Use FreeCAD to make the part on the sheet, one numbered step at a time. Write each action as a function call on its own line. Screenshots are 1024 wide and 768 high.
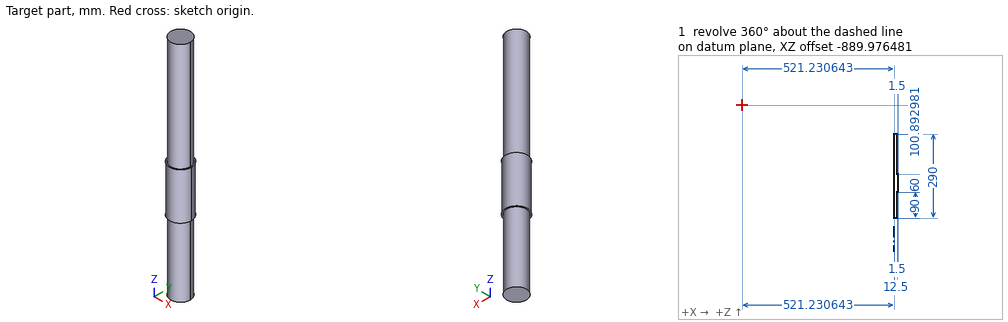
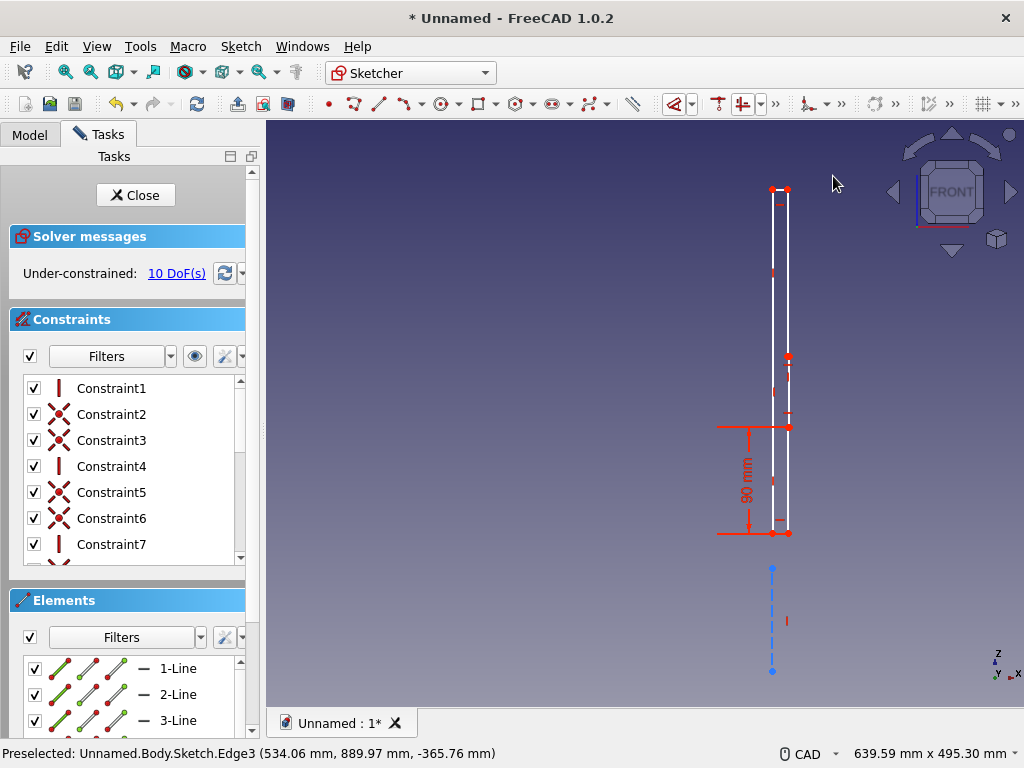
click(789, 399)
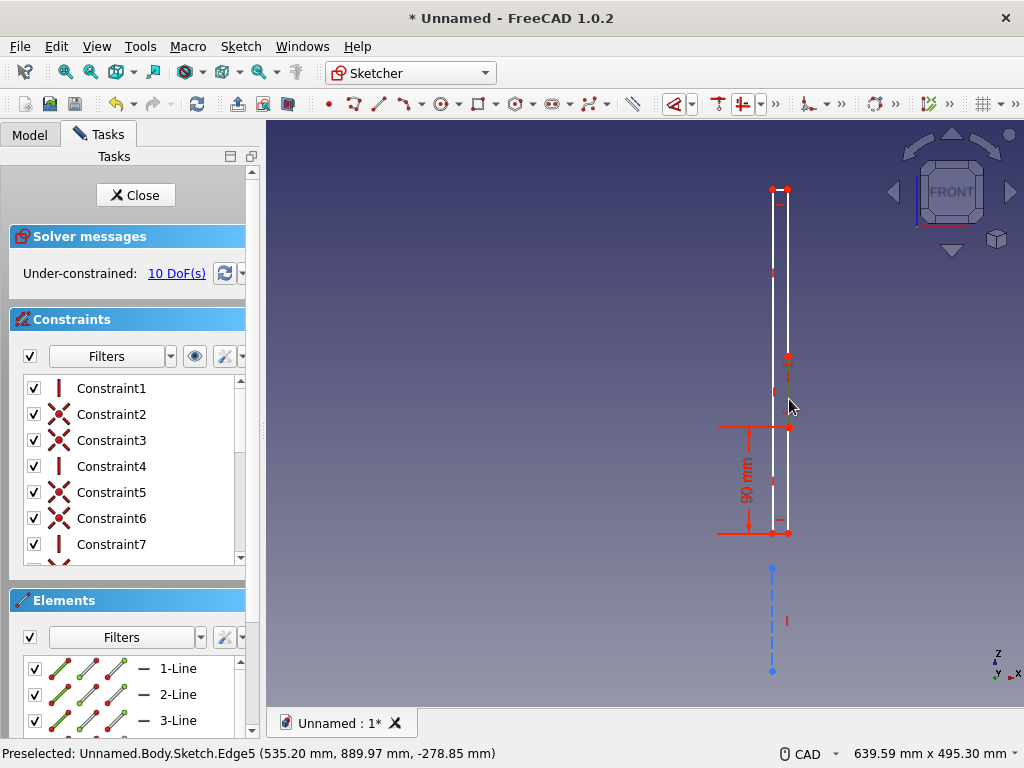
key(i)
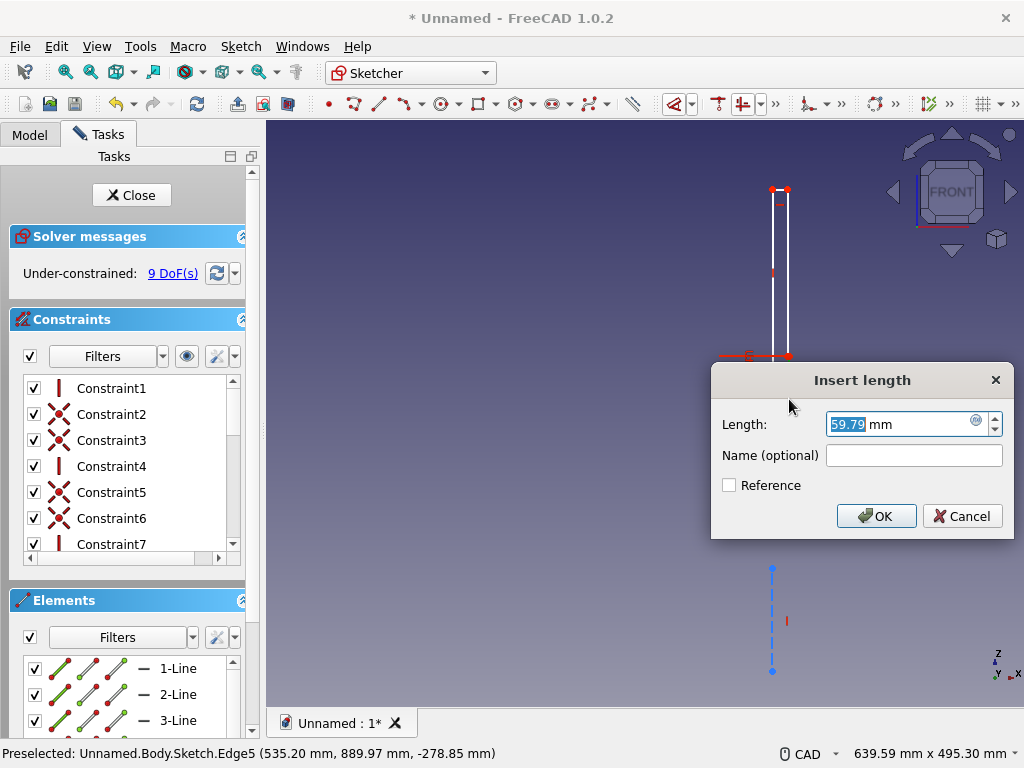
text(60)
key(Return)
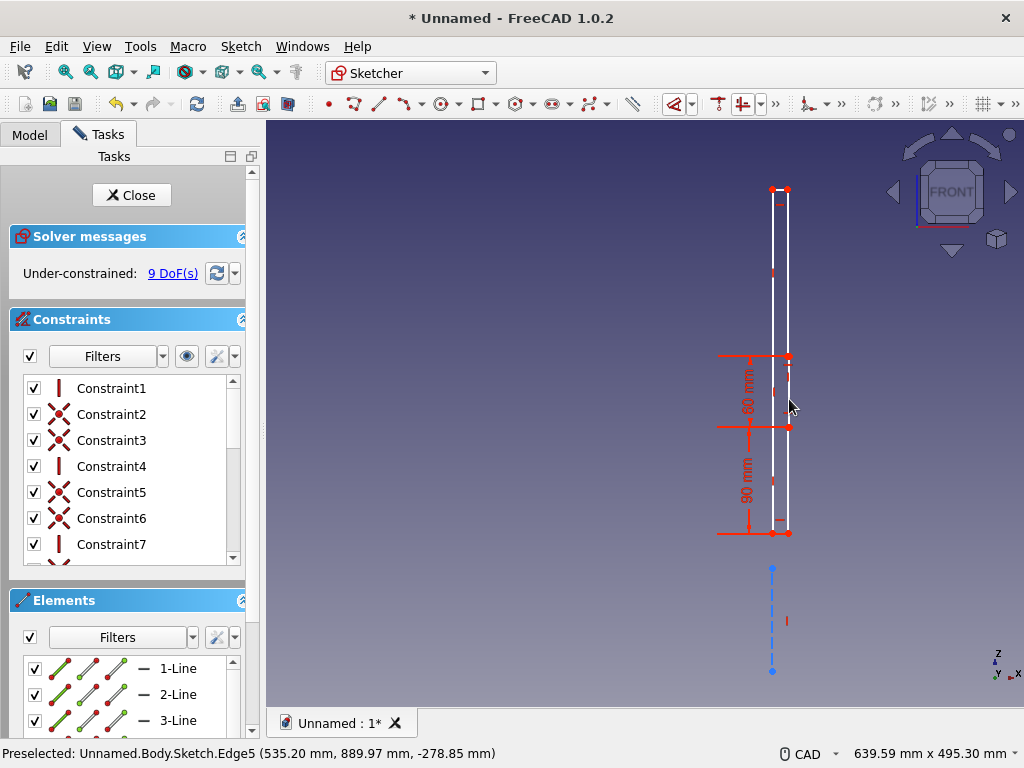
click(773, 293)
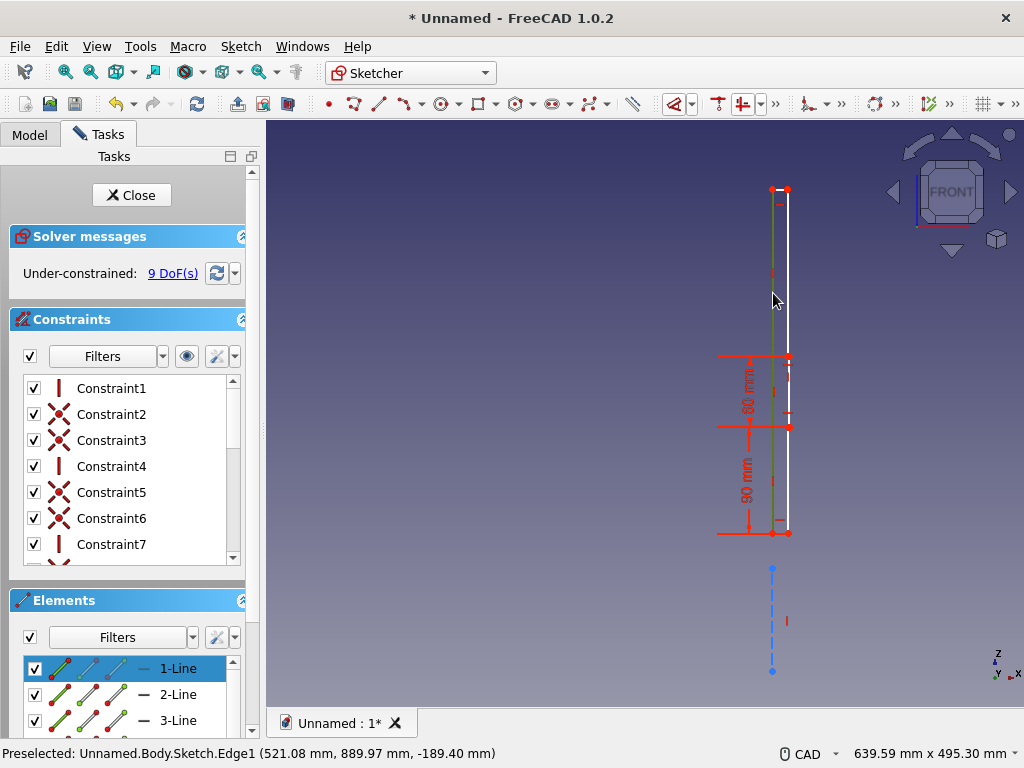
key(i)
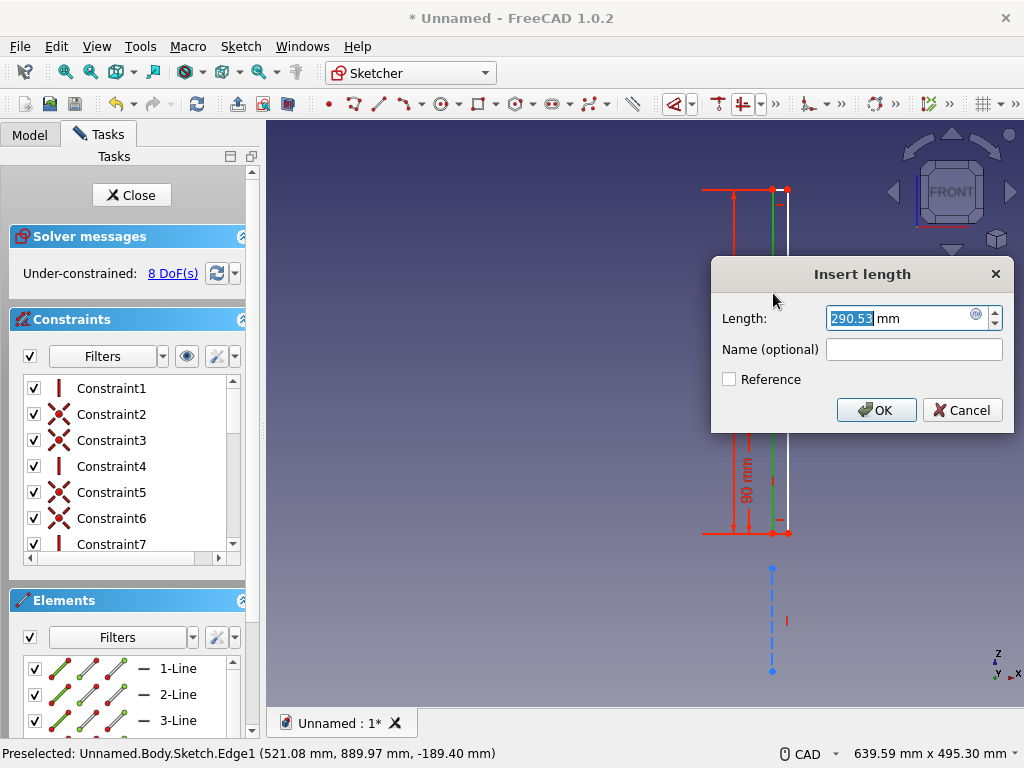
text(290)
key(Return)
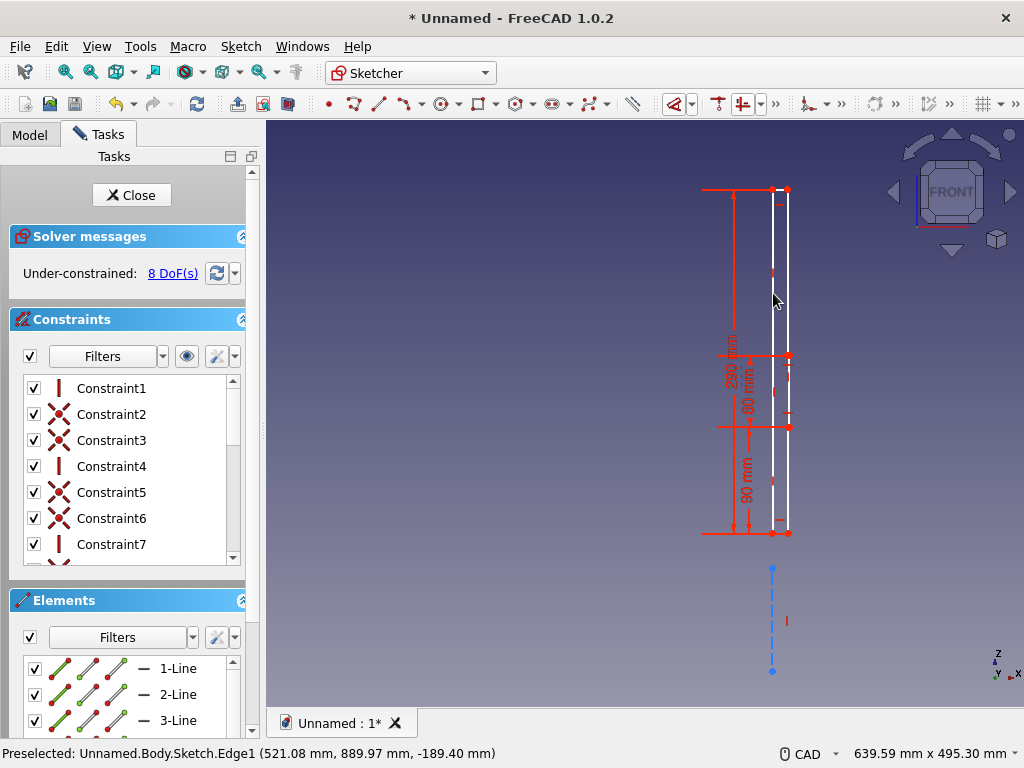
scroll(789, 427, up, 16)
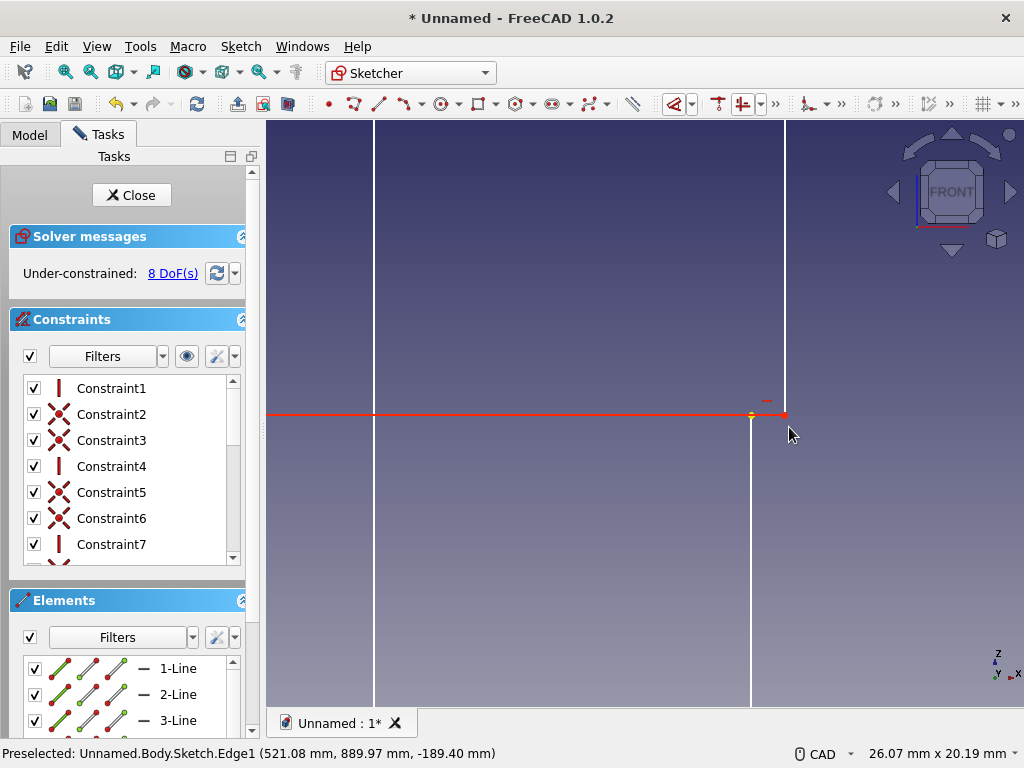
click(768, 415)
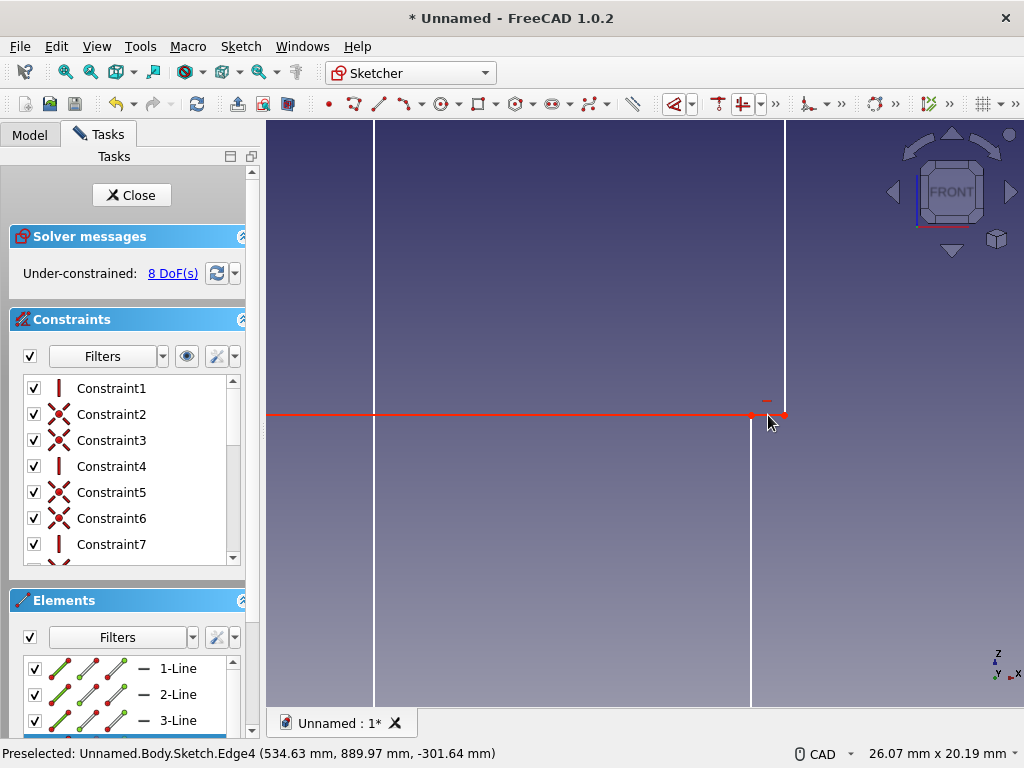
click(692, 104)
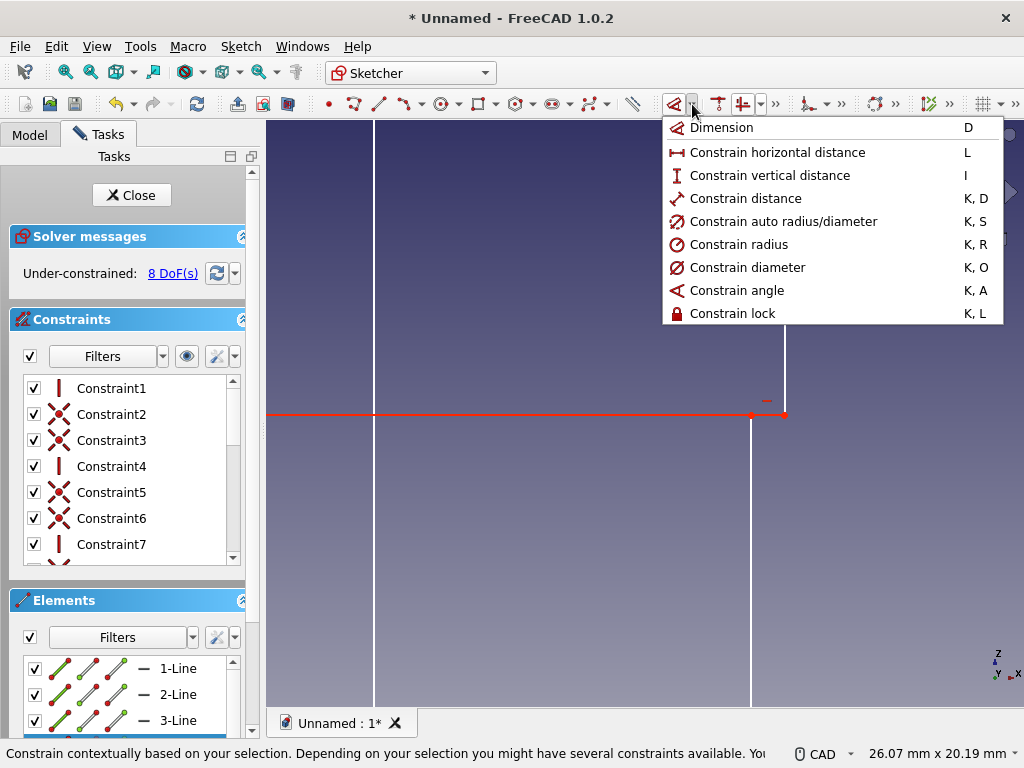
click(833, 152)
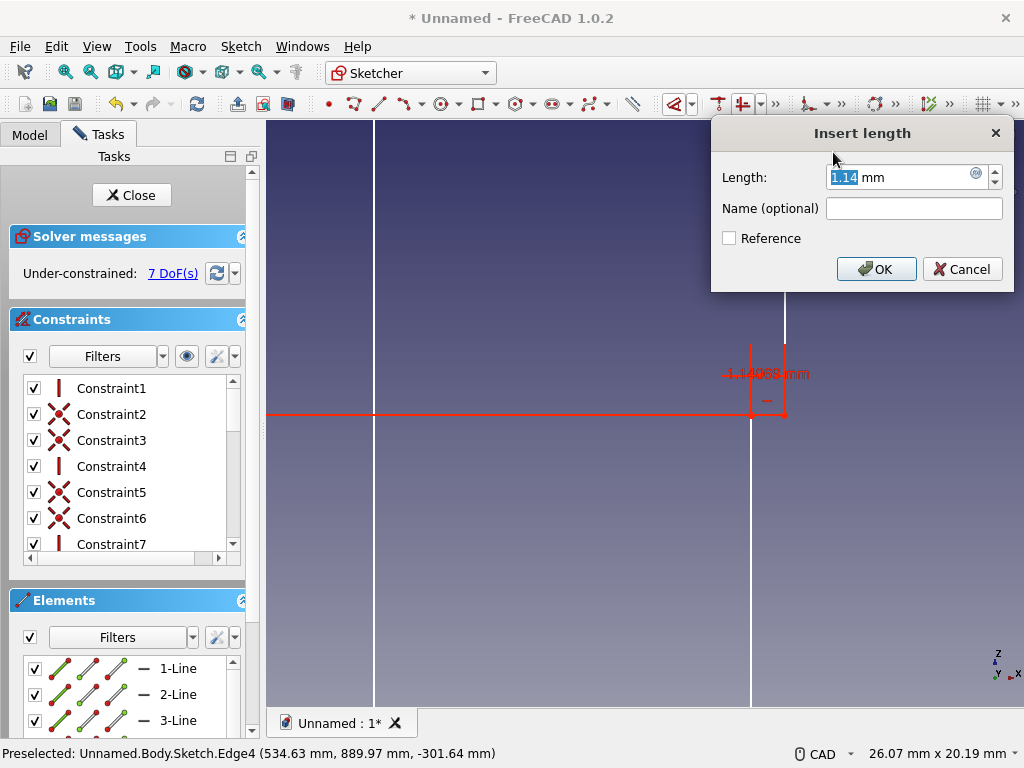
text(1.5)
key(Return)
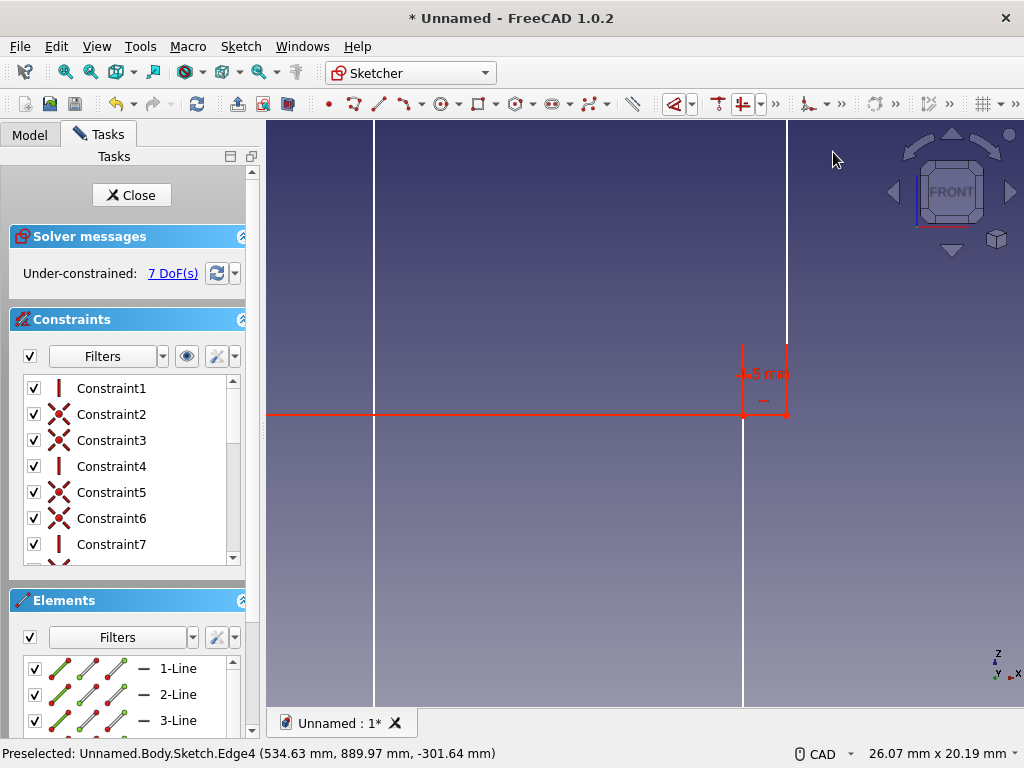
scroll(789, 453, down, 18)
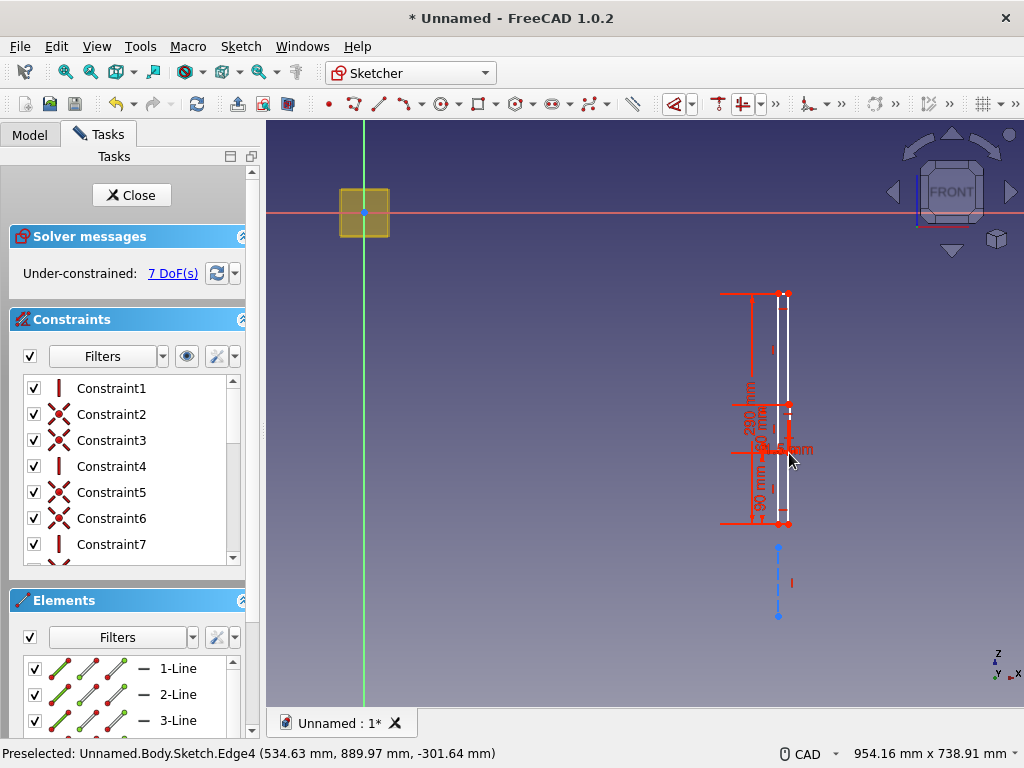
scroll(789, 405, up, 18)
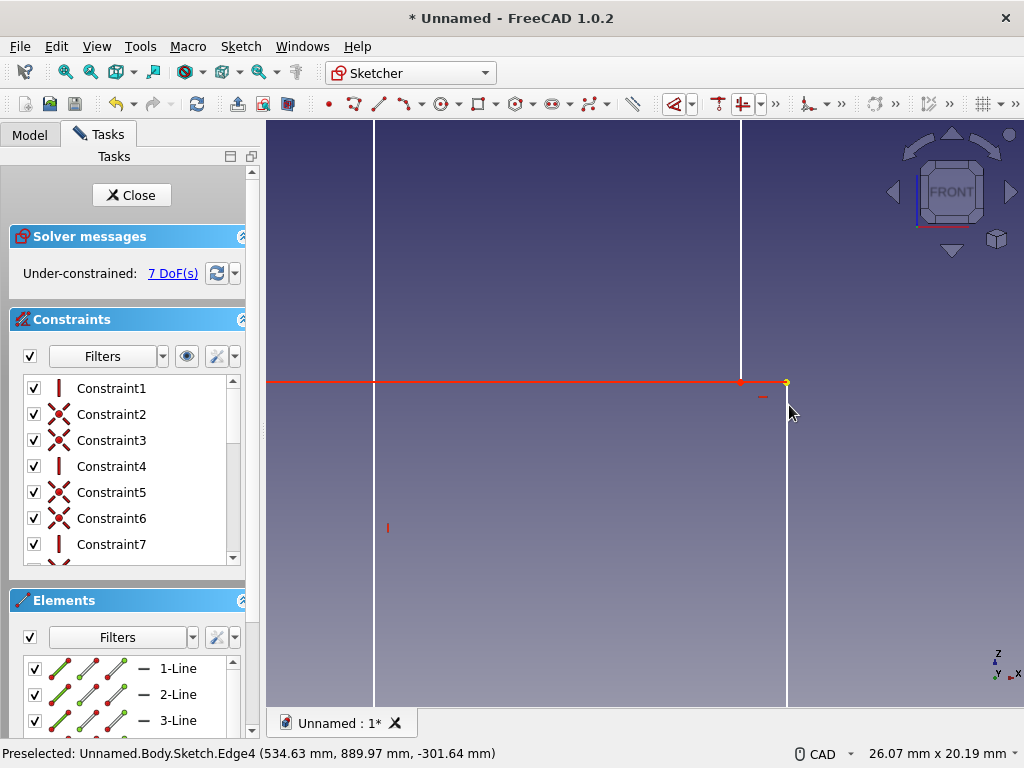
click(773, 382)